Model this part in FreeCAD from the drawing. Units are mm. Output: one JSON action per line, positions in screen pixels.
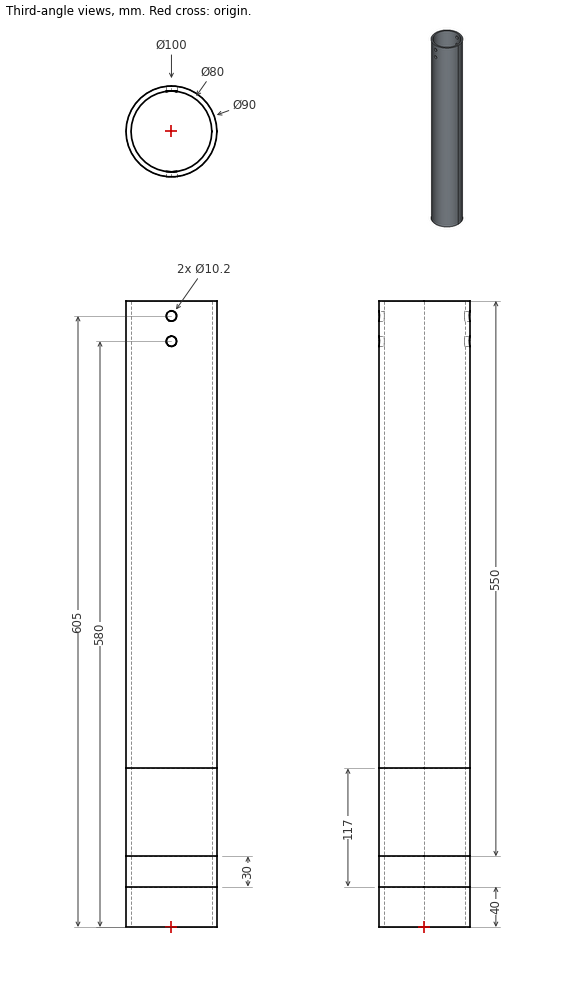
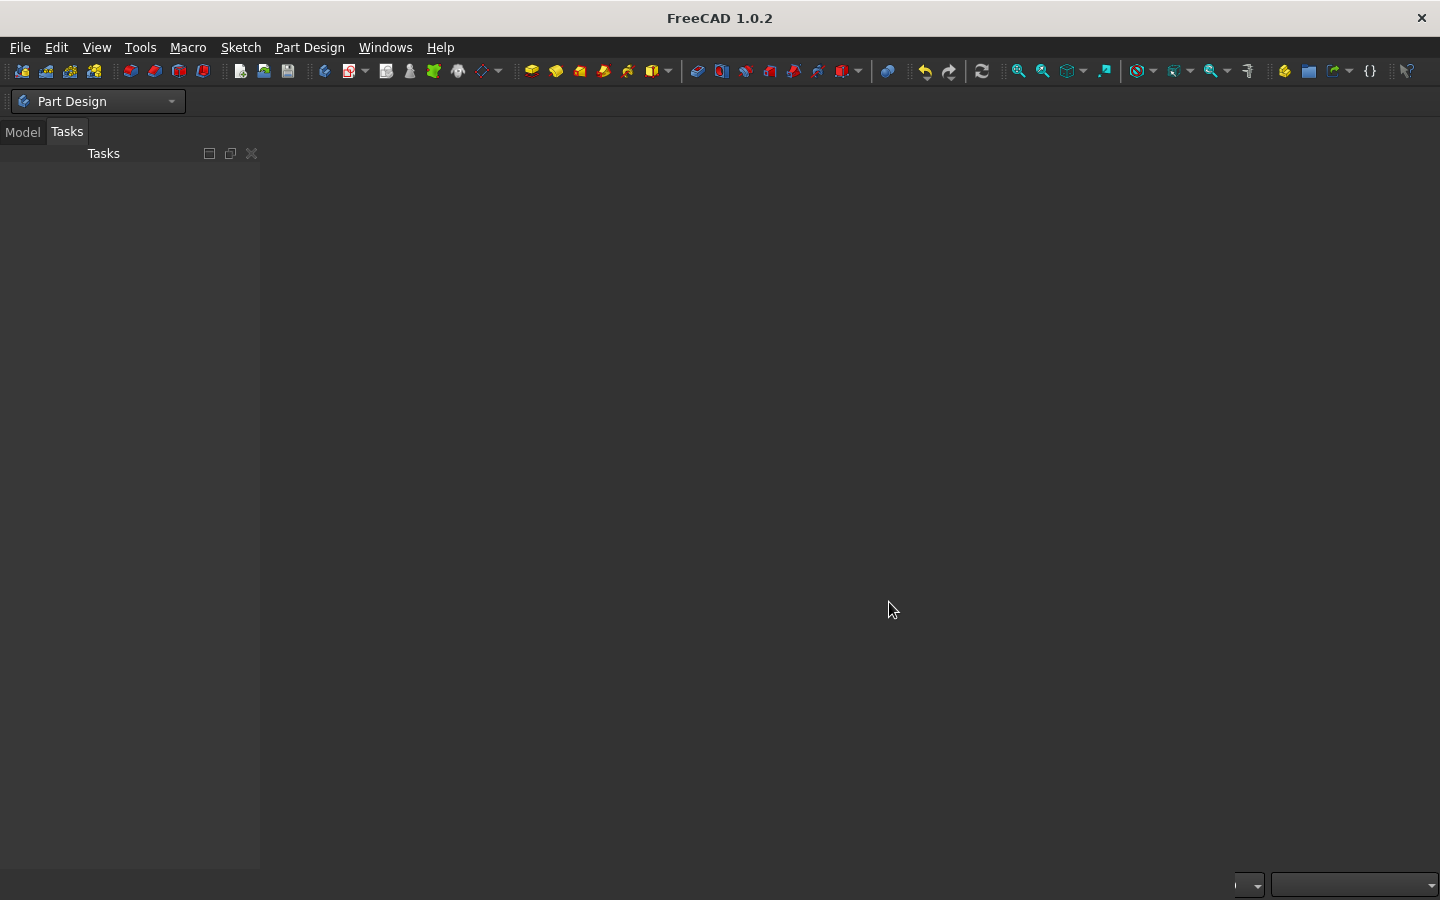
{"action": "key", "text": "ctrl+n"}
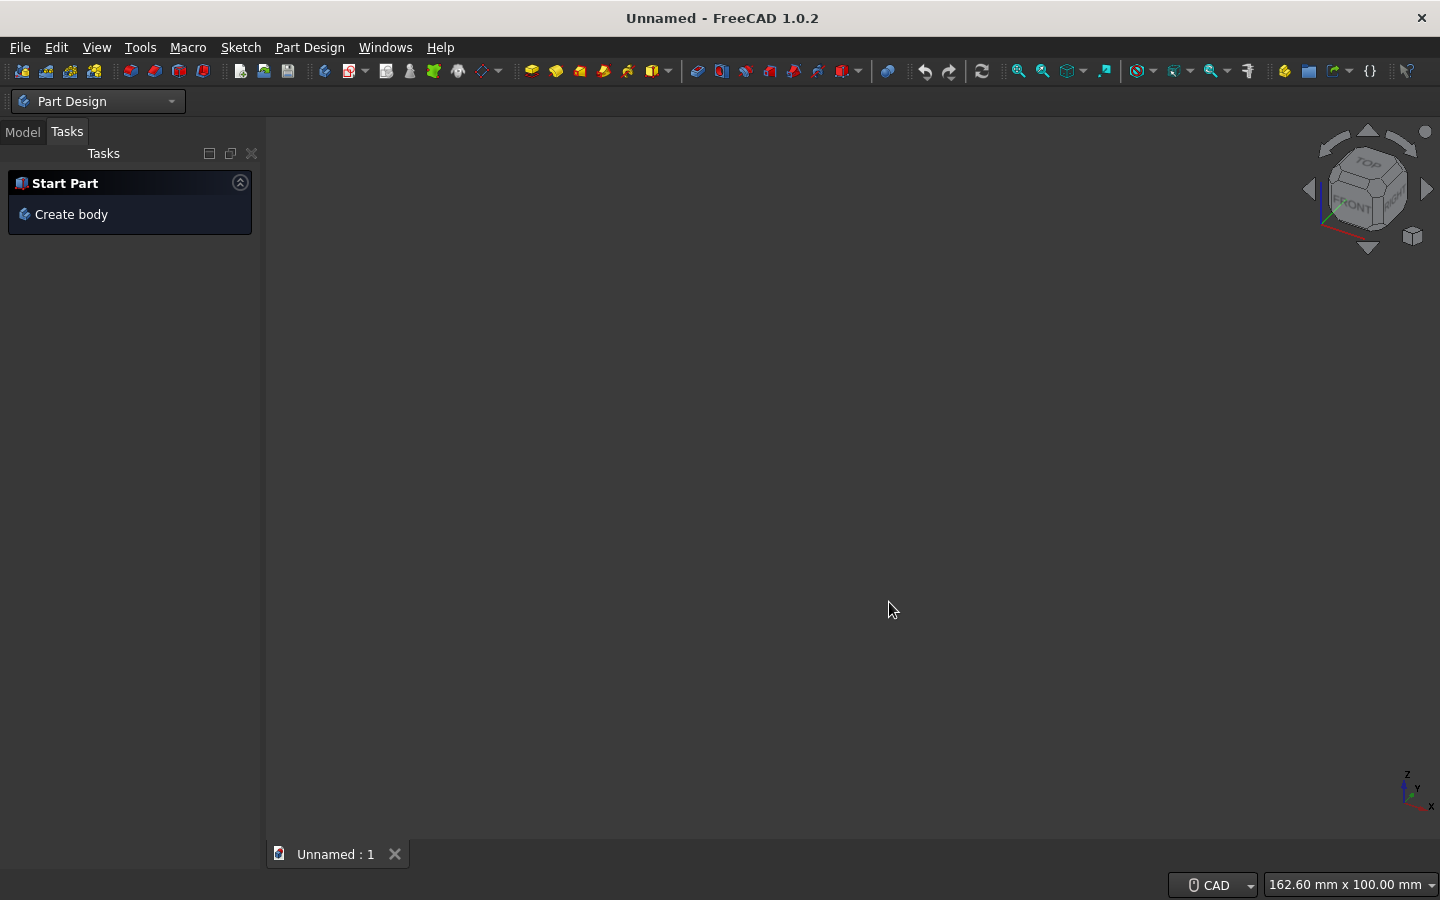
{"action": "left_click", "coordinate": [350, 72]}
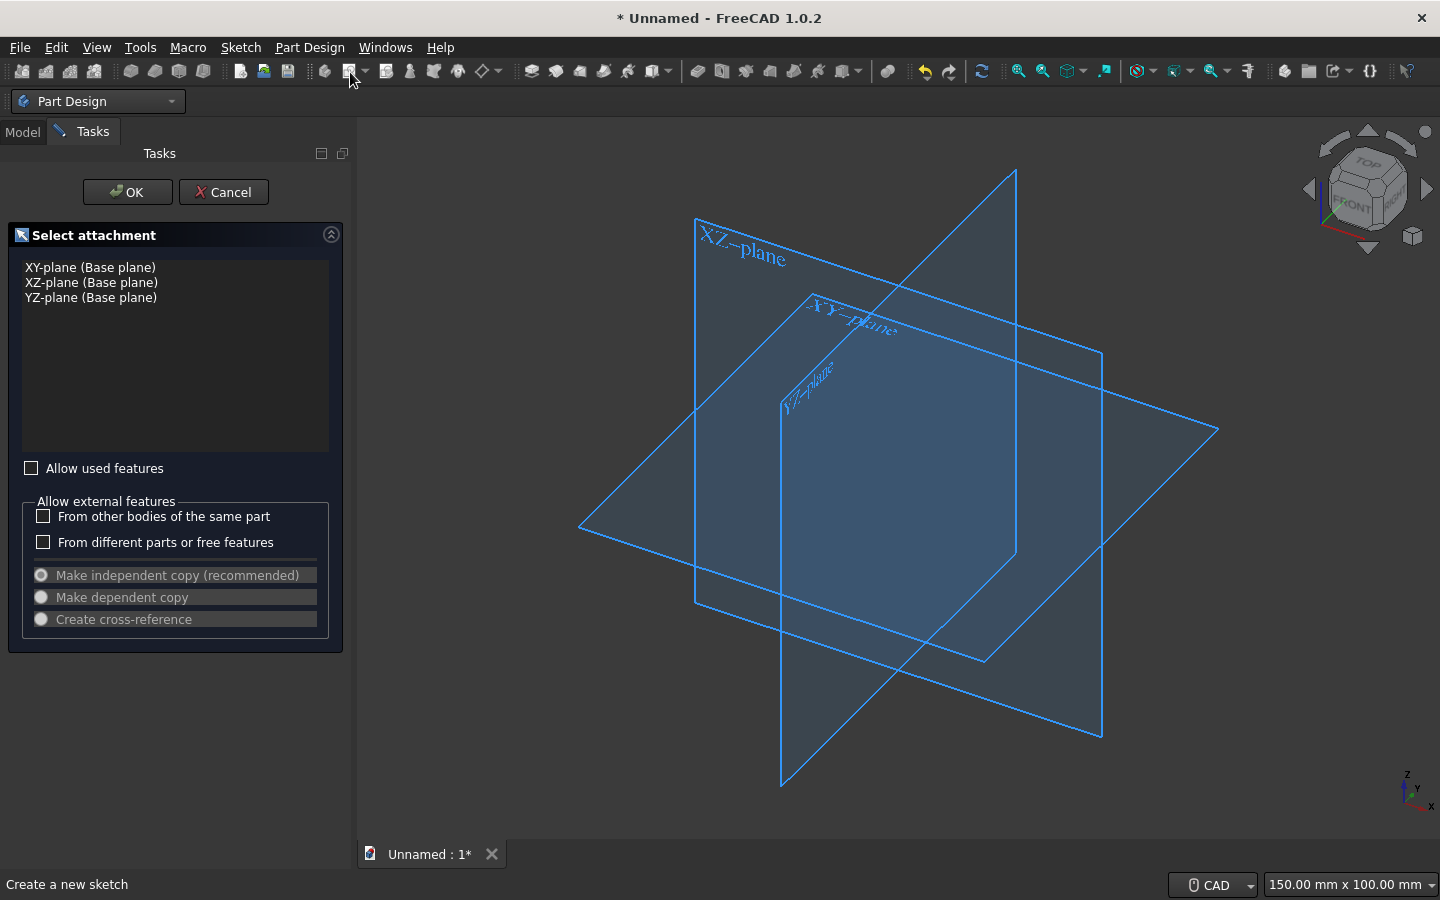
{"action": "left_click", "coordinate": [82, 268]}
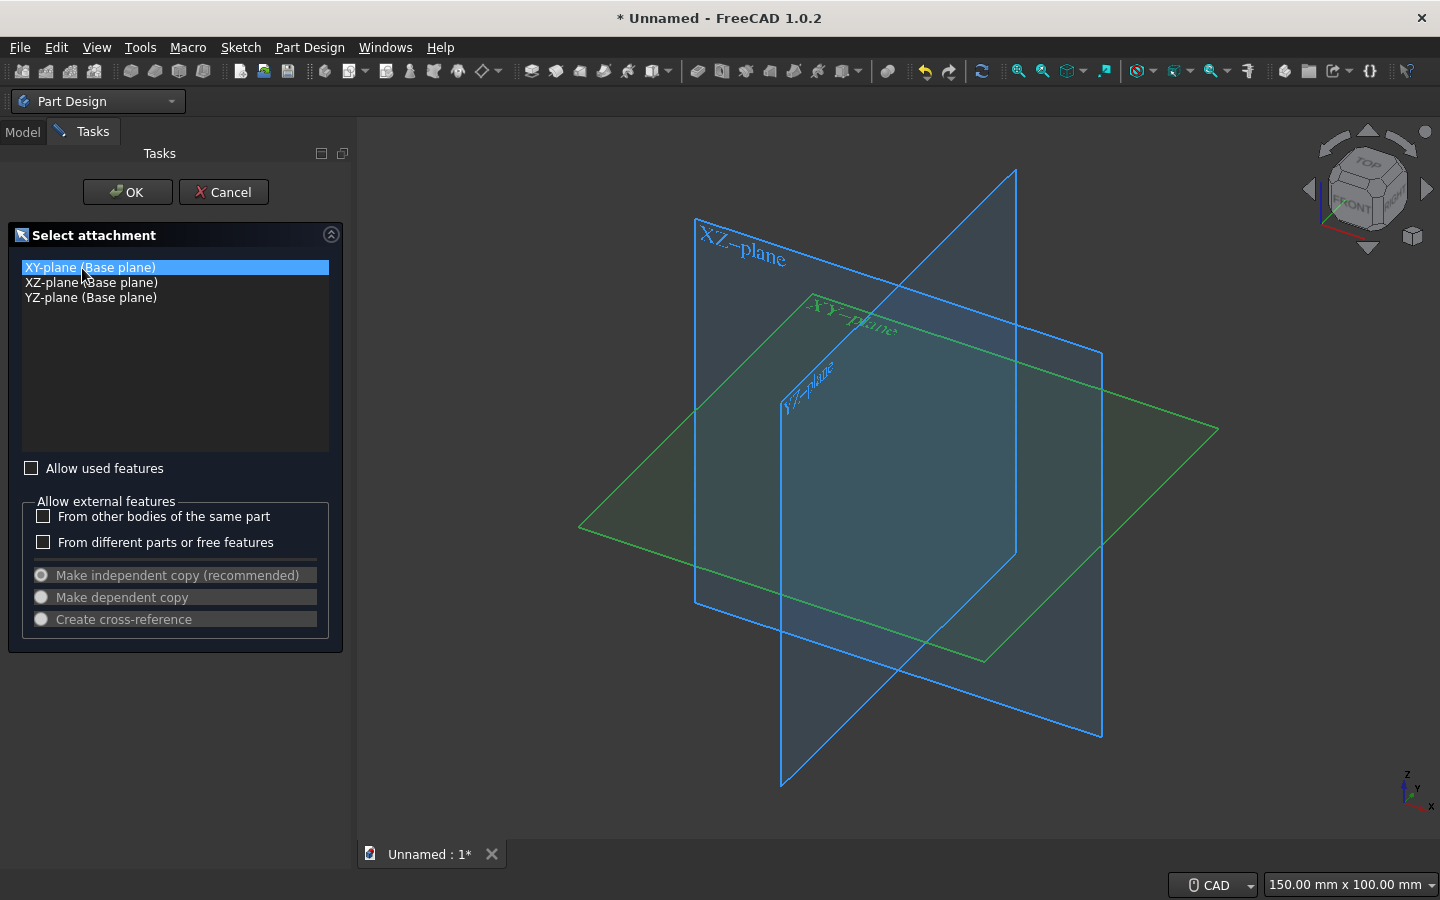
{"action": "left_click", "coordinate": [128, 192]}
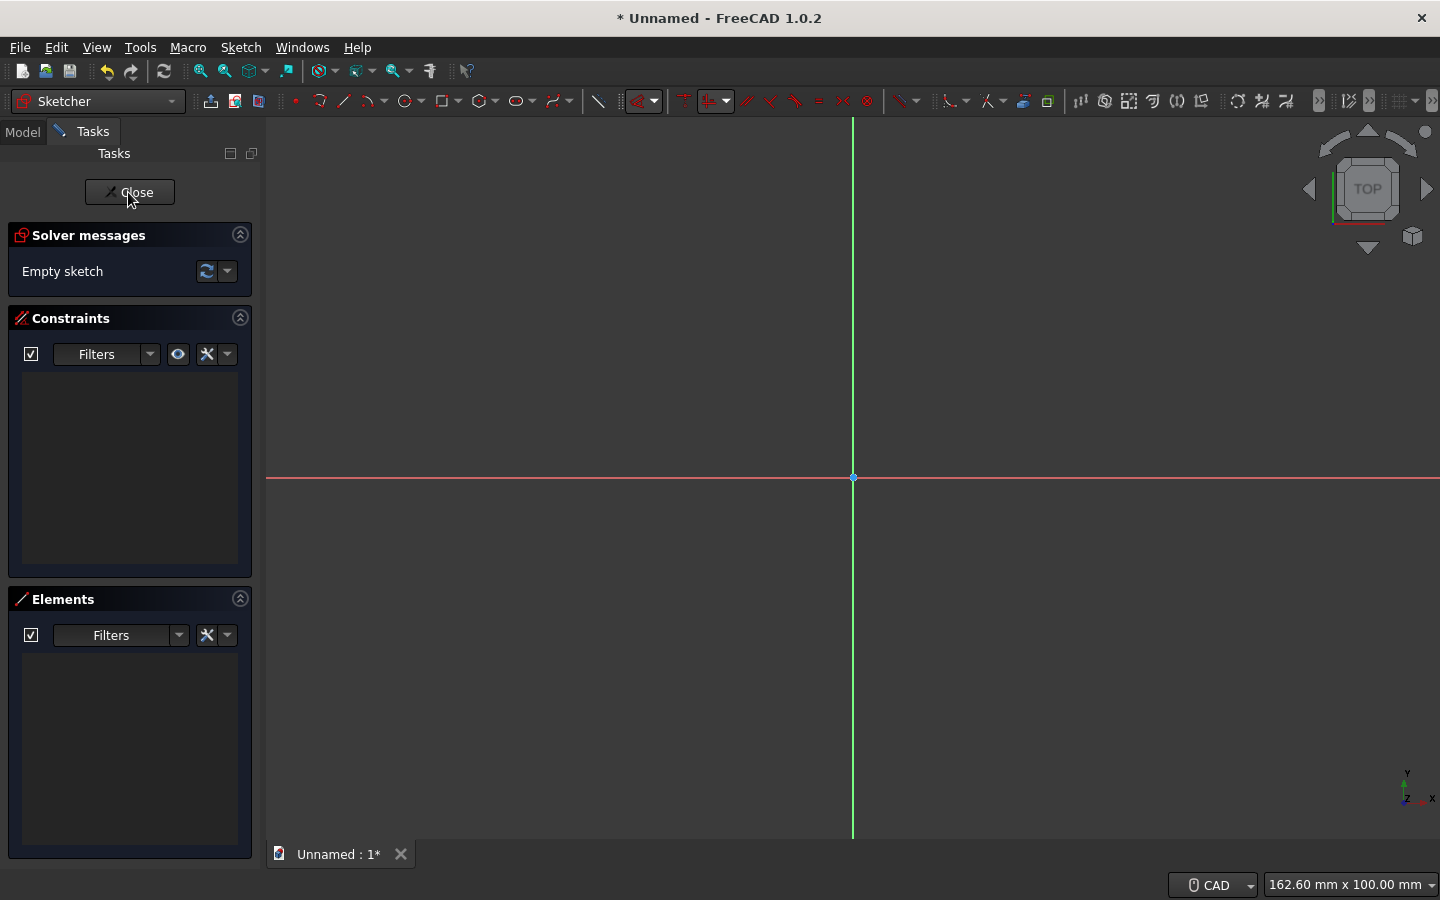
{"action": "scroll", "coordinate": [645, 478], "scroll_direction": "down", "scroll_amount": 2}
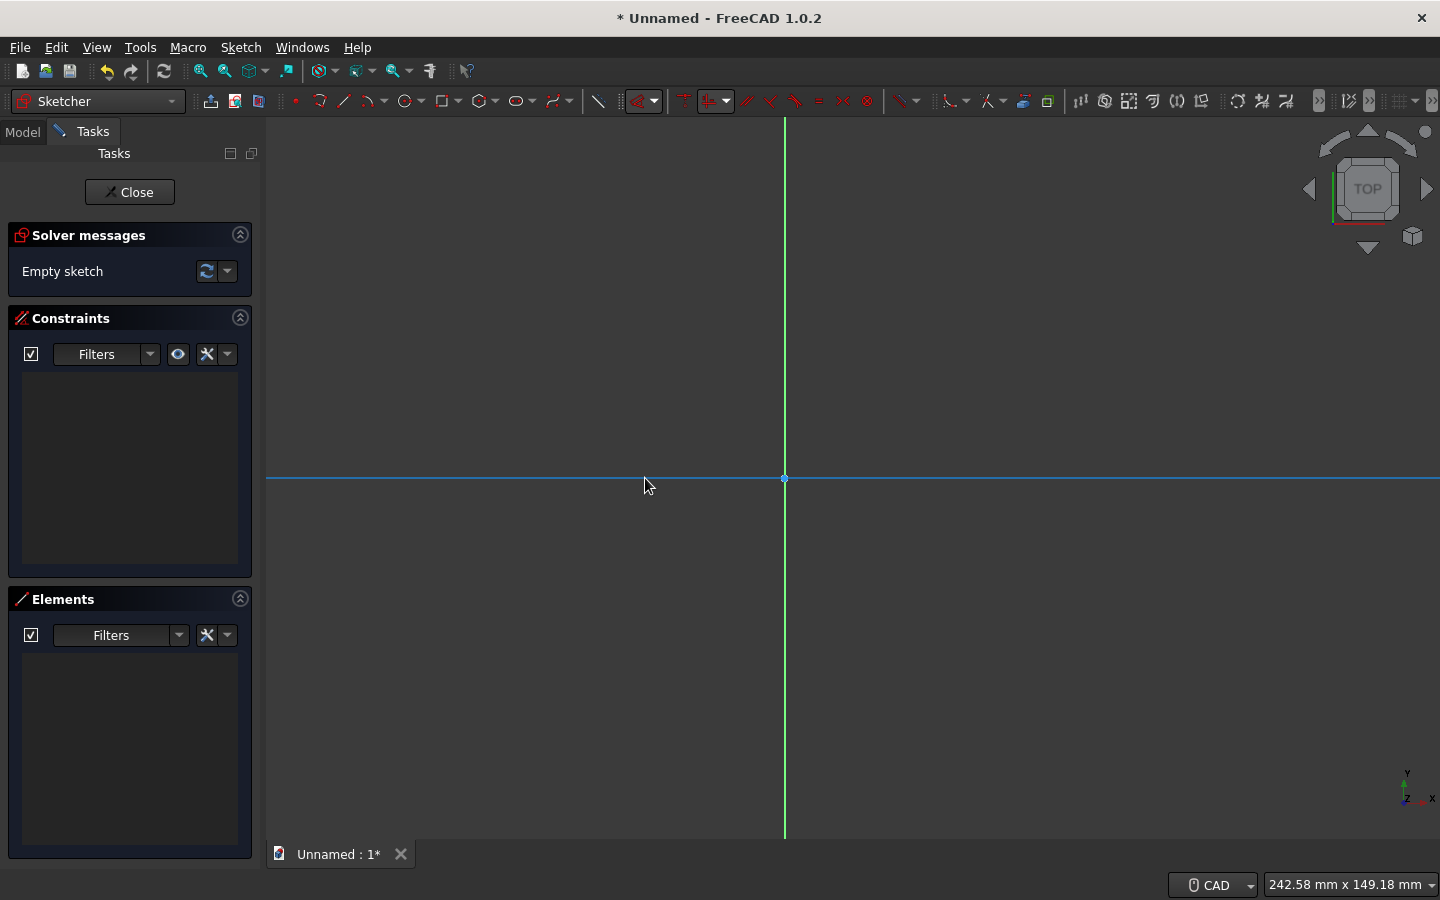
{"action": "key", "text": "g c"}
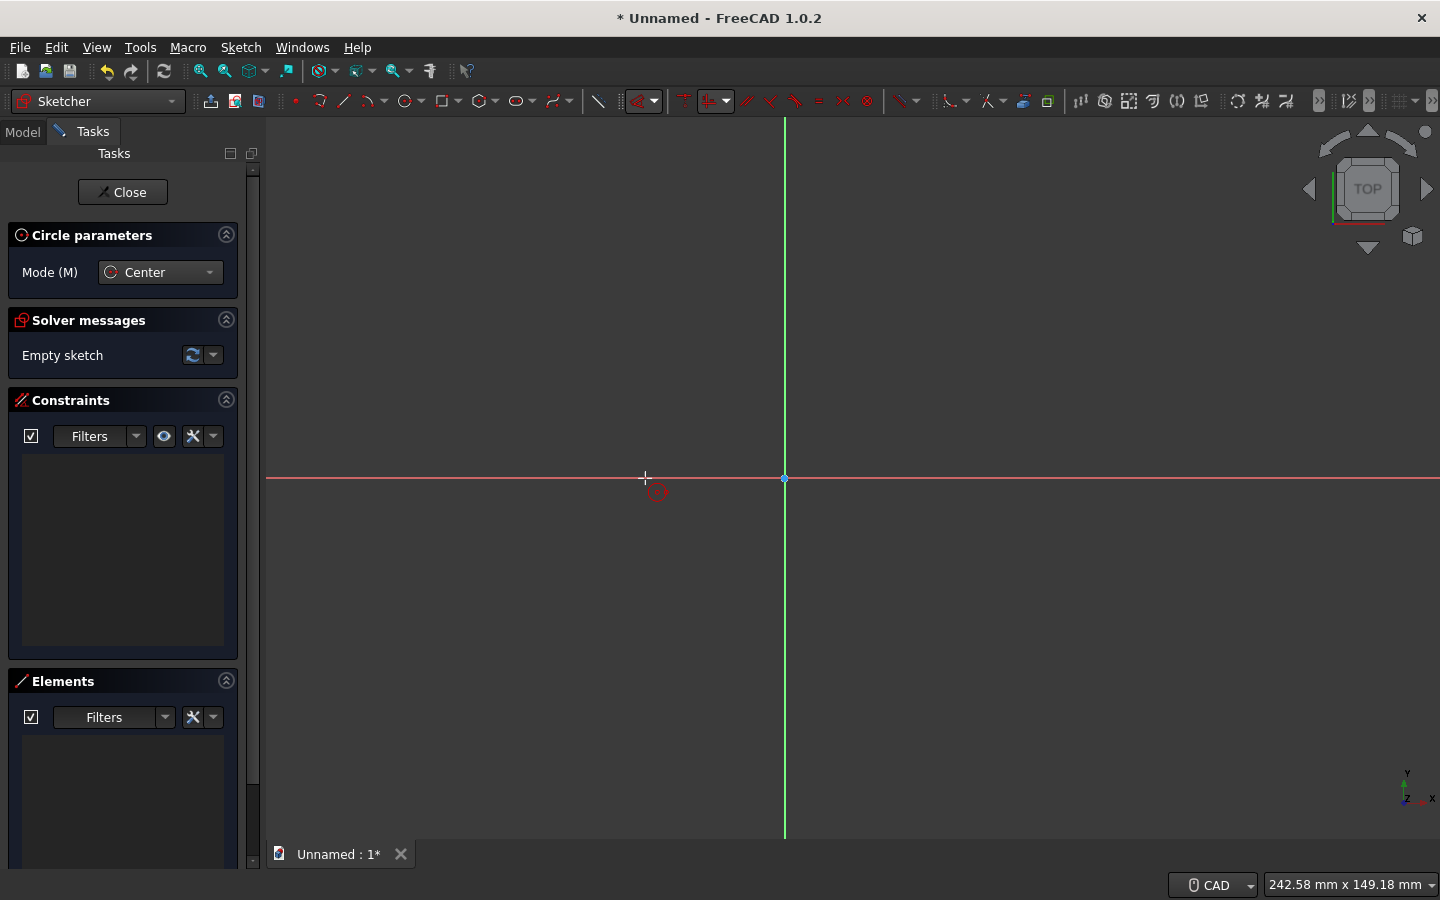
{"action": "left_click", "coordinate": [785, 478]}
{"action": "mouse_move", "coordinate": [939, 324]}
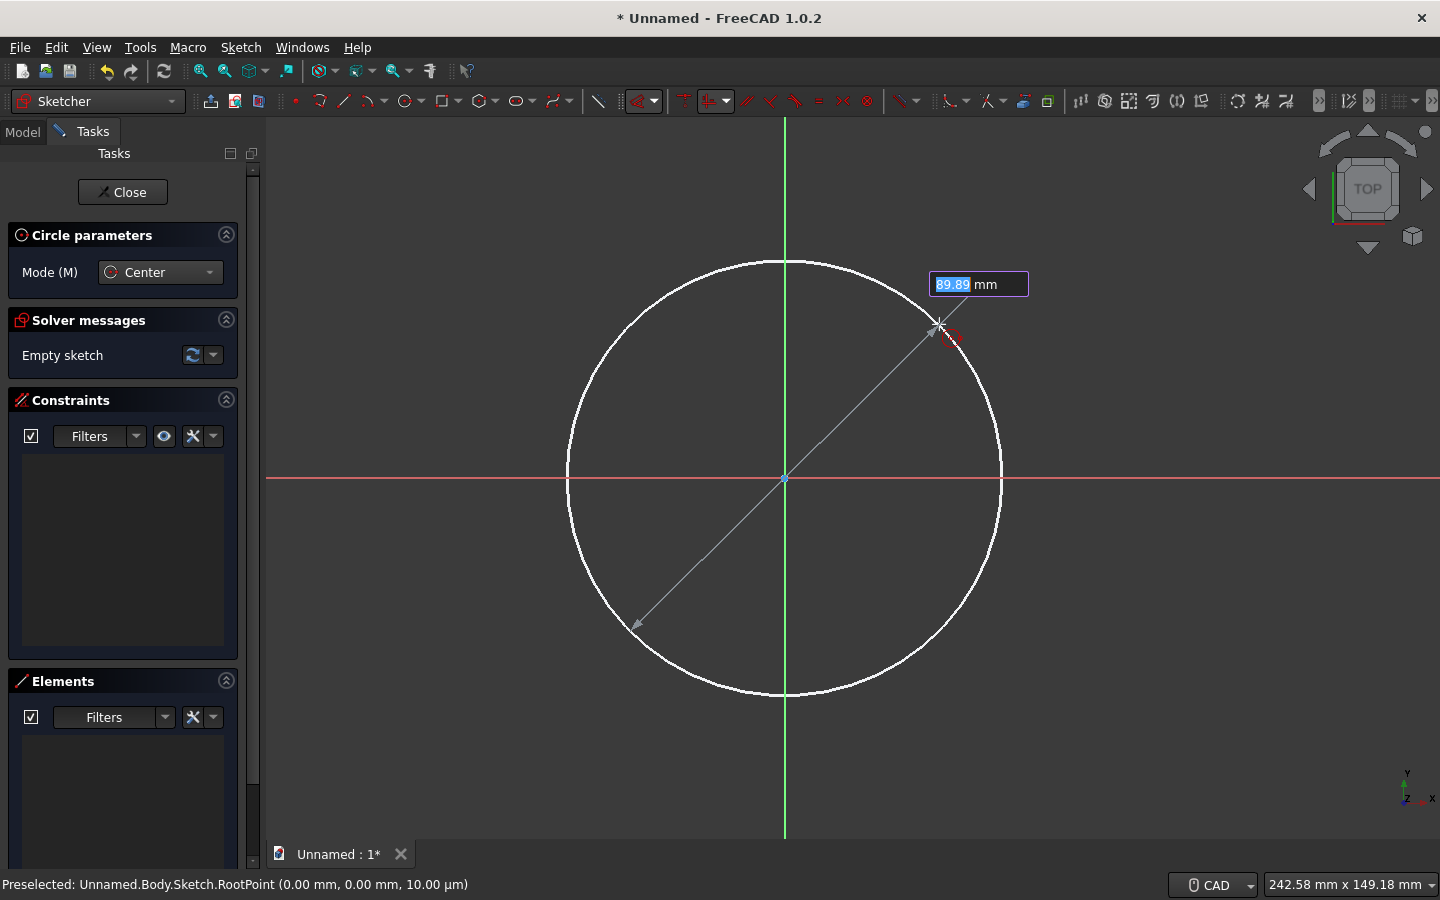
{"action": "type", "text": "90"}
{"action": "key", "text": "Return"}